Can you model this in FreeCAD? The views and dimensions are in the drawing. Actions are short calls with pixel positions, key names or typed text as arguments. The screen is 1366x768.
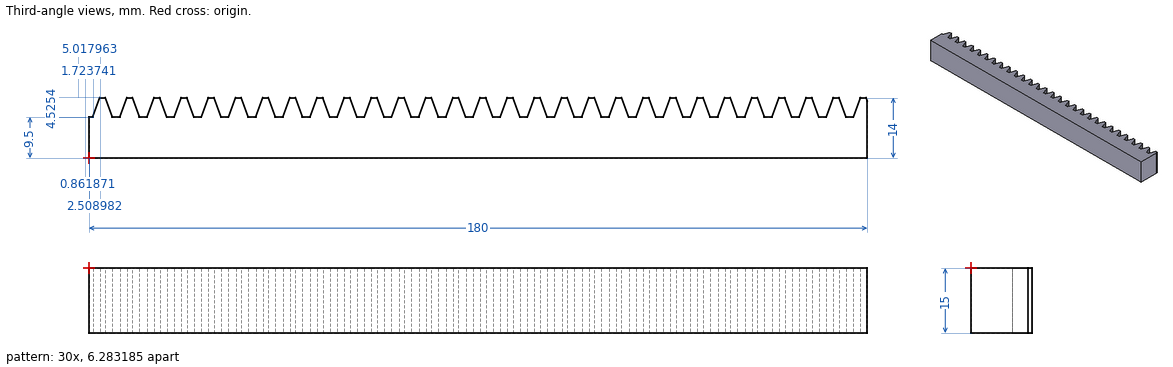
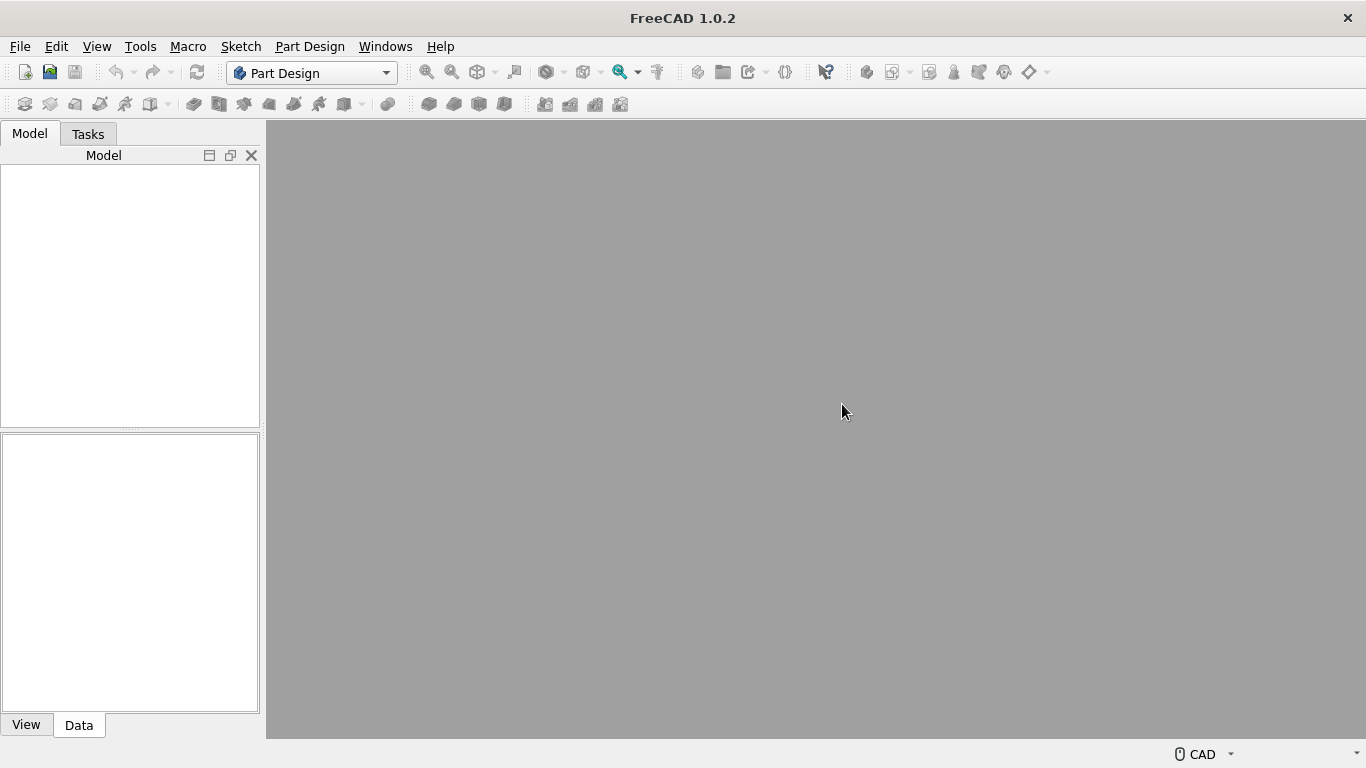
key(ctrl+n)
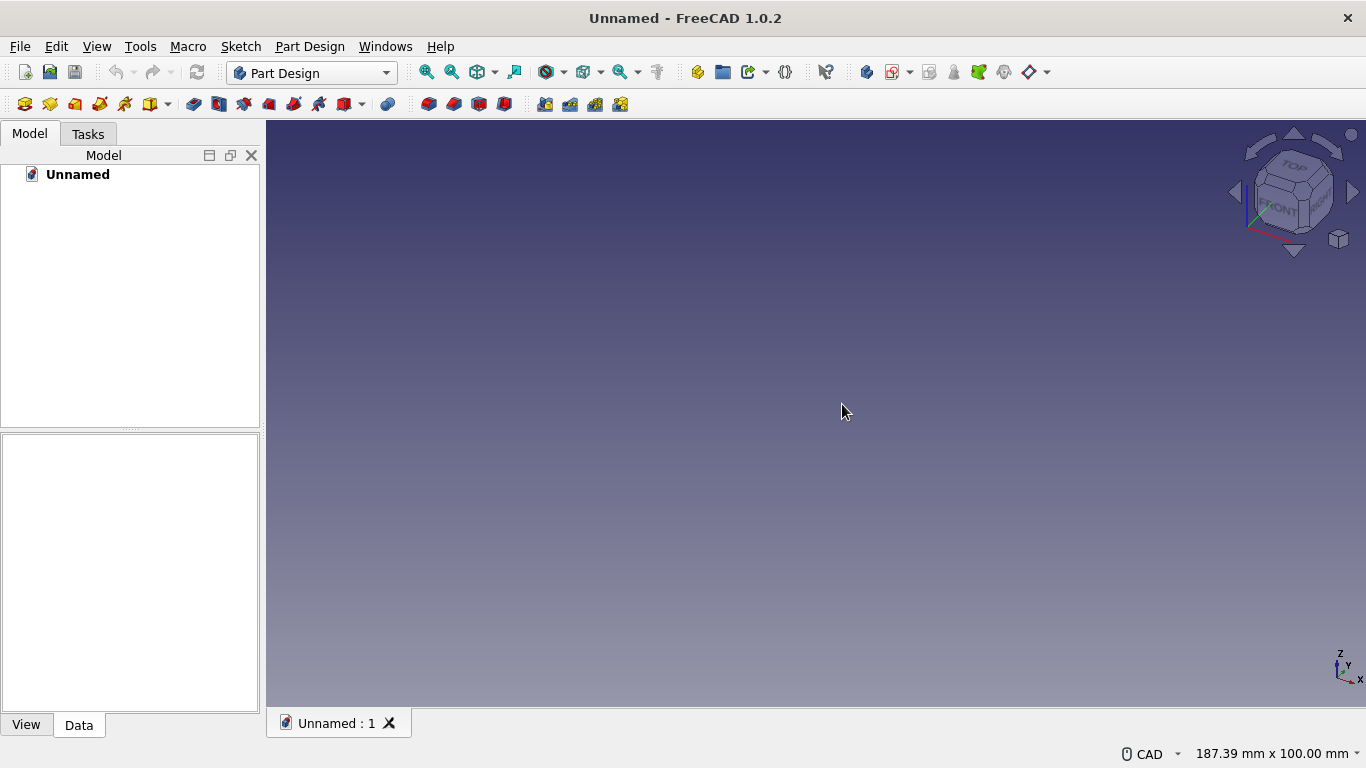
click(892, 72)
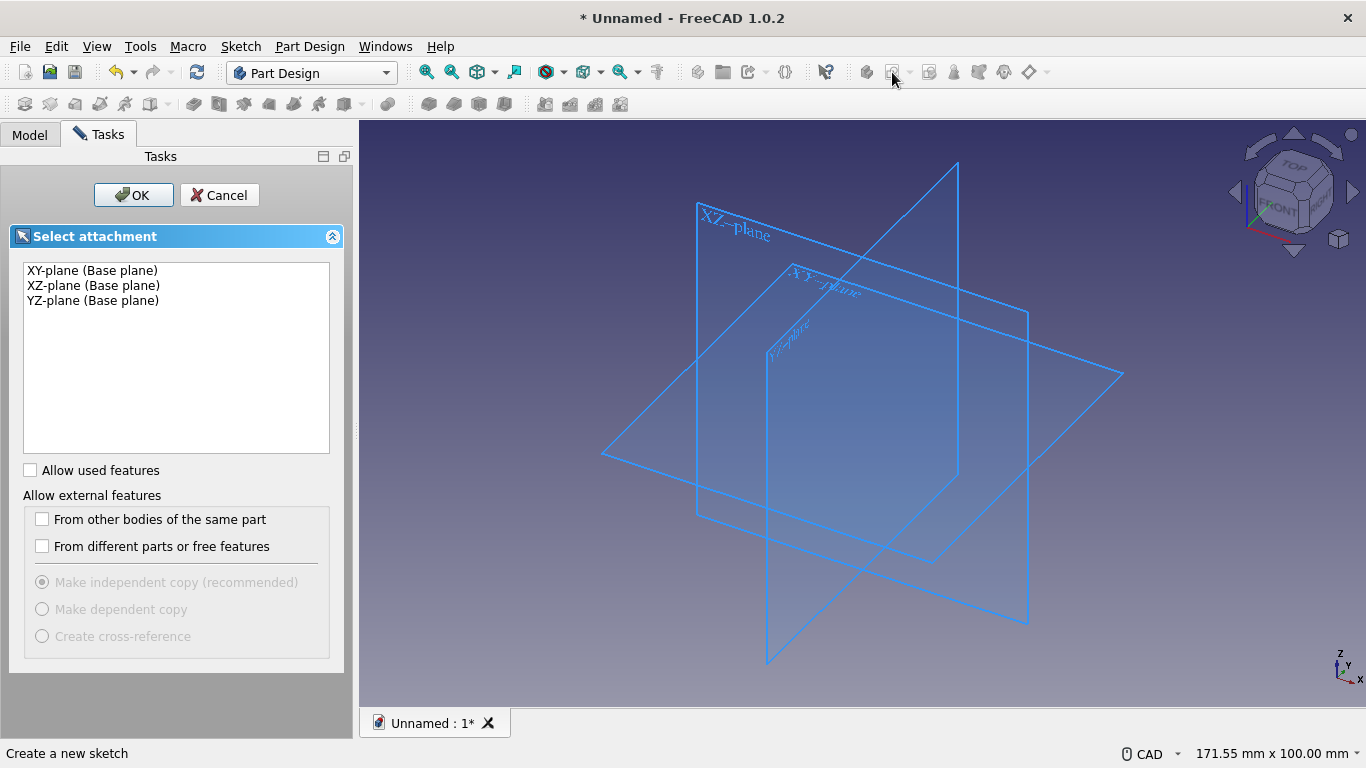
click(84, 270)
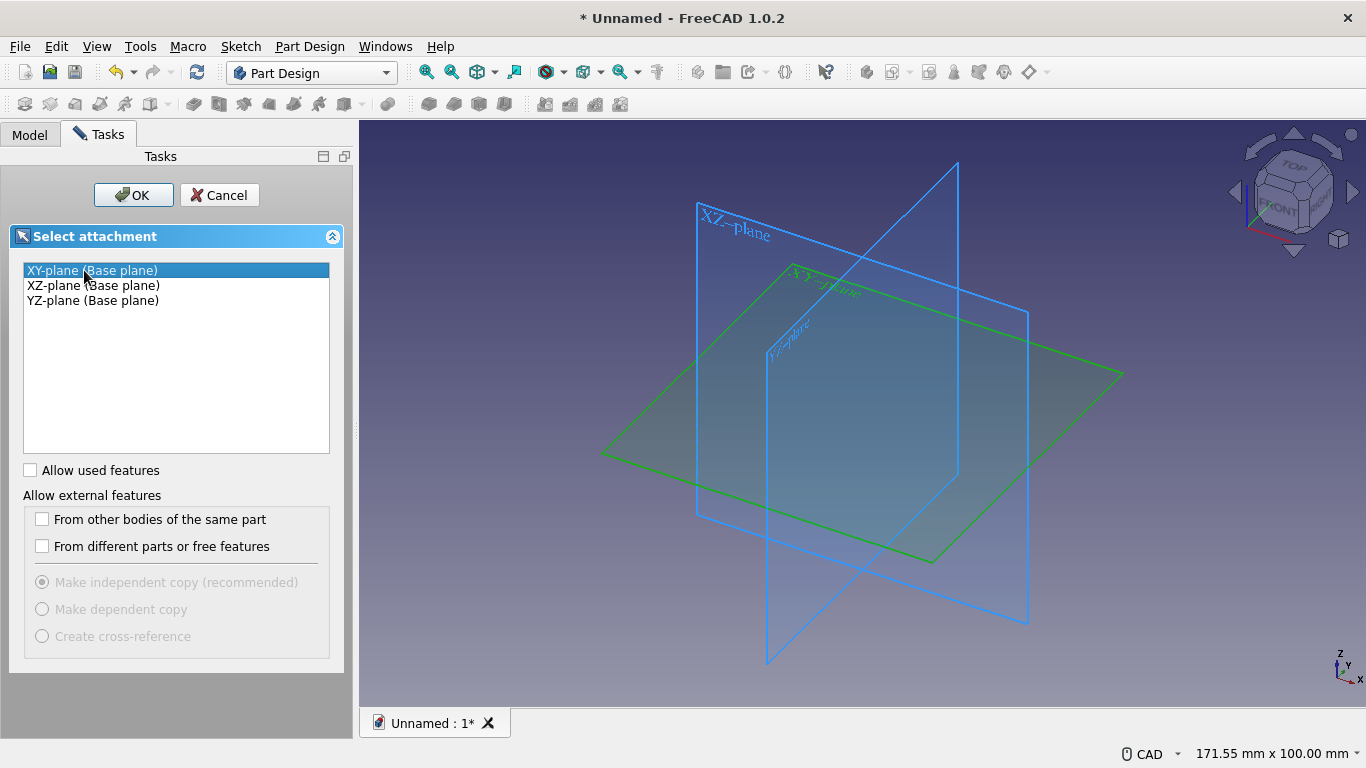
click(134, 195)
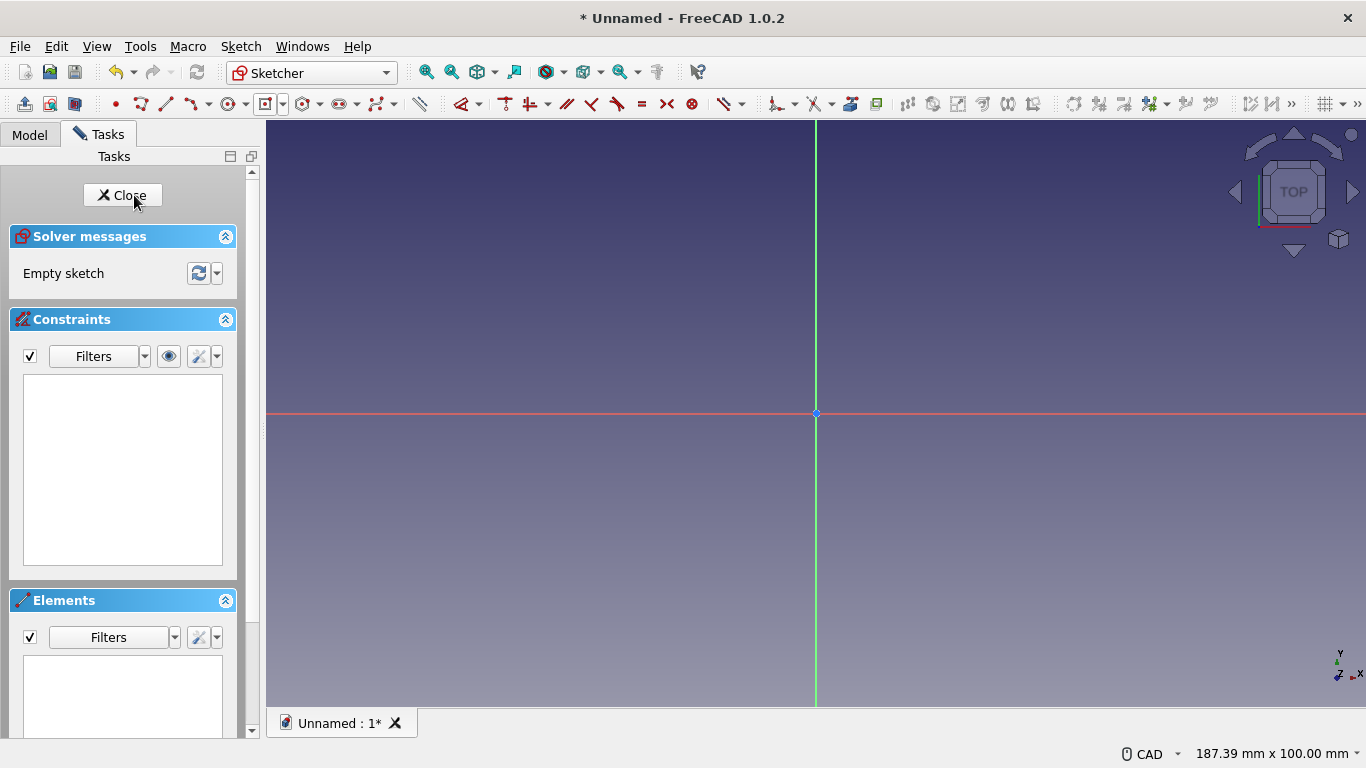
scroll(294, 463, down, 3)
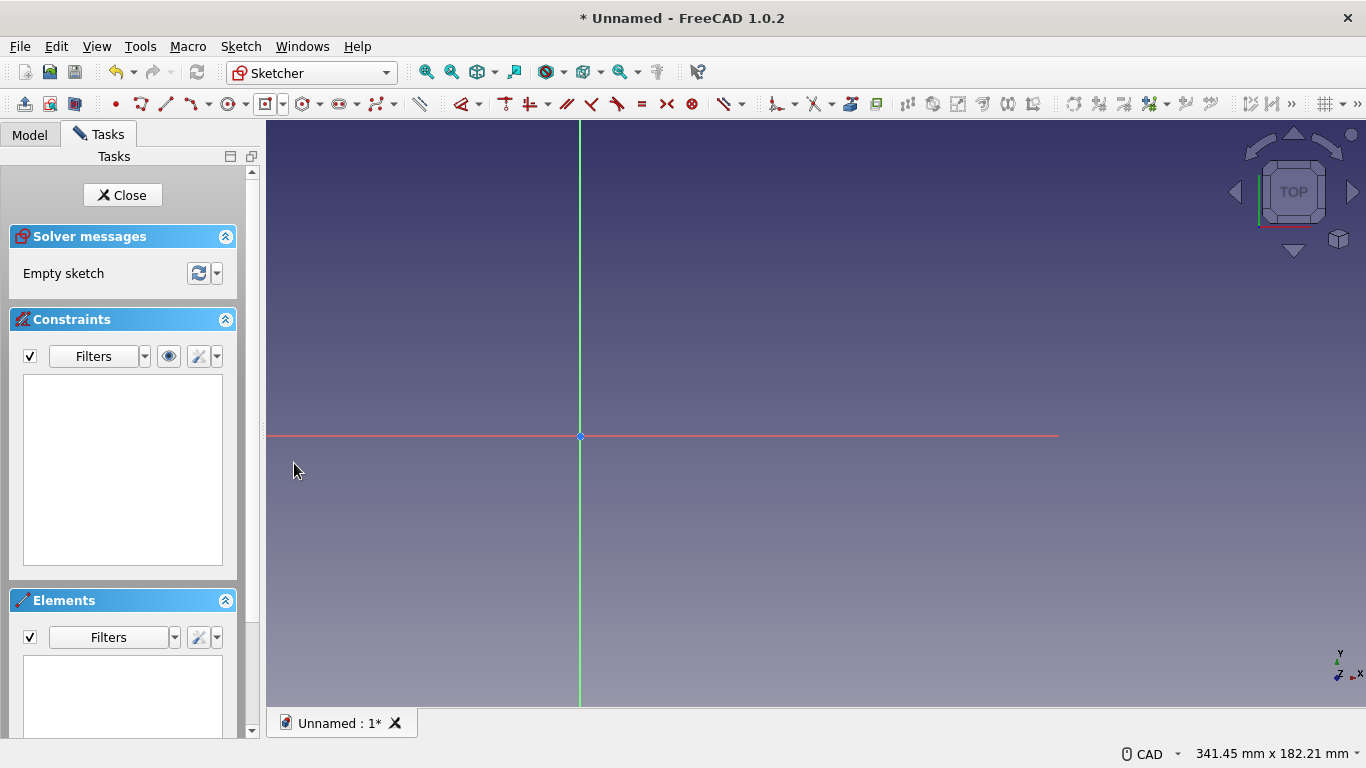
key(g)
key(r)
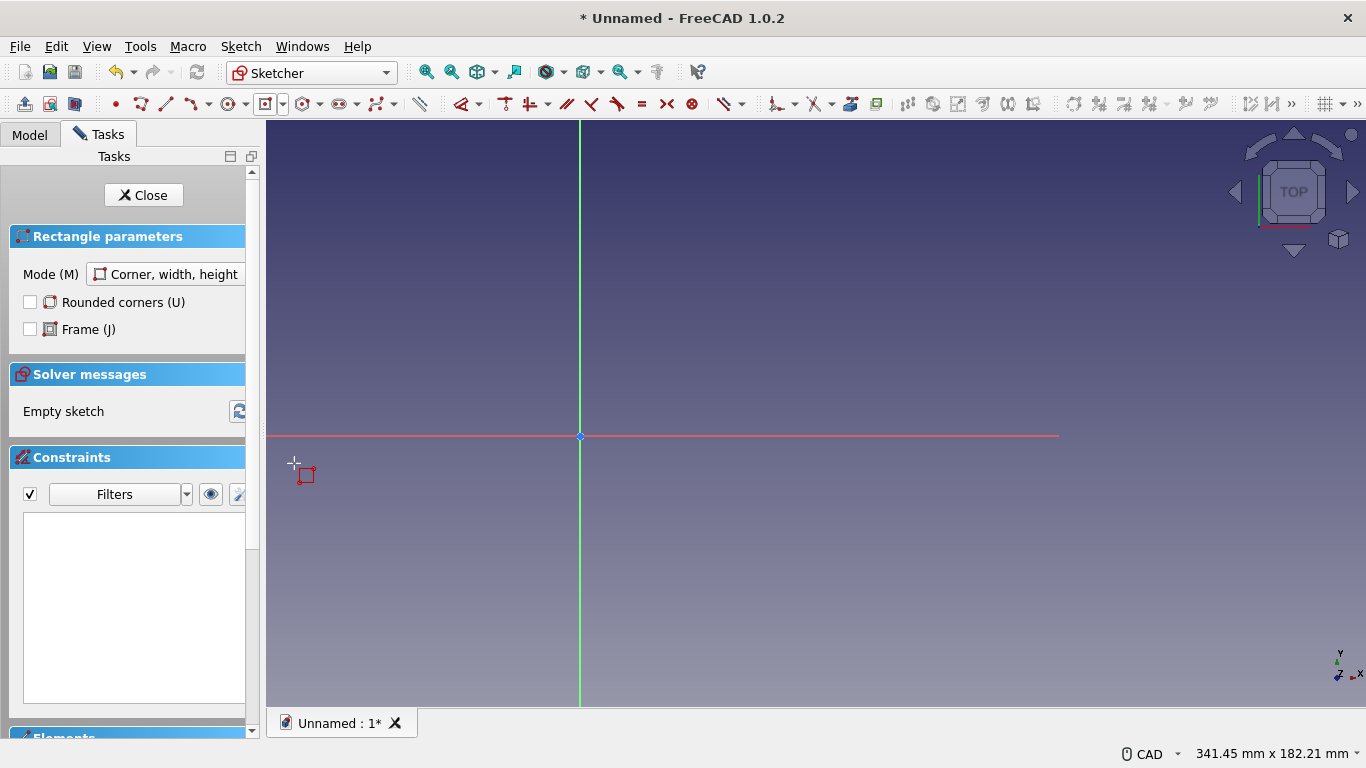
click(580, 436)
move(1160, 391)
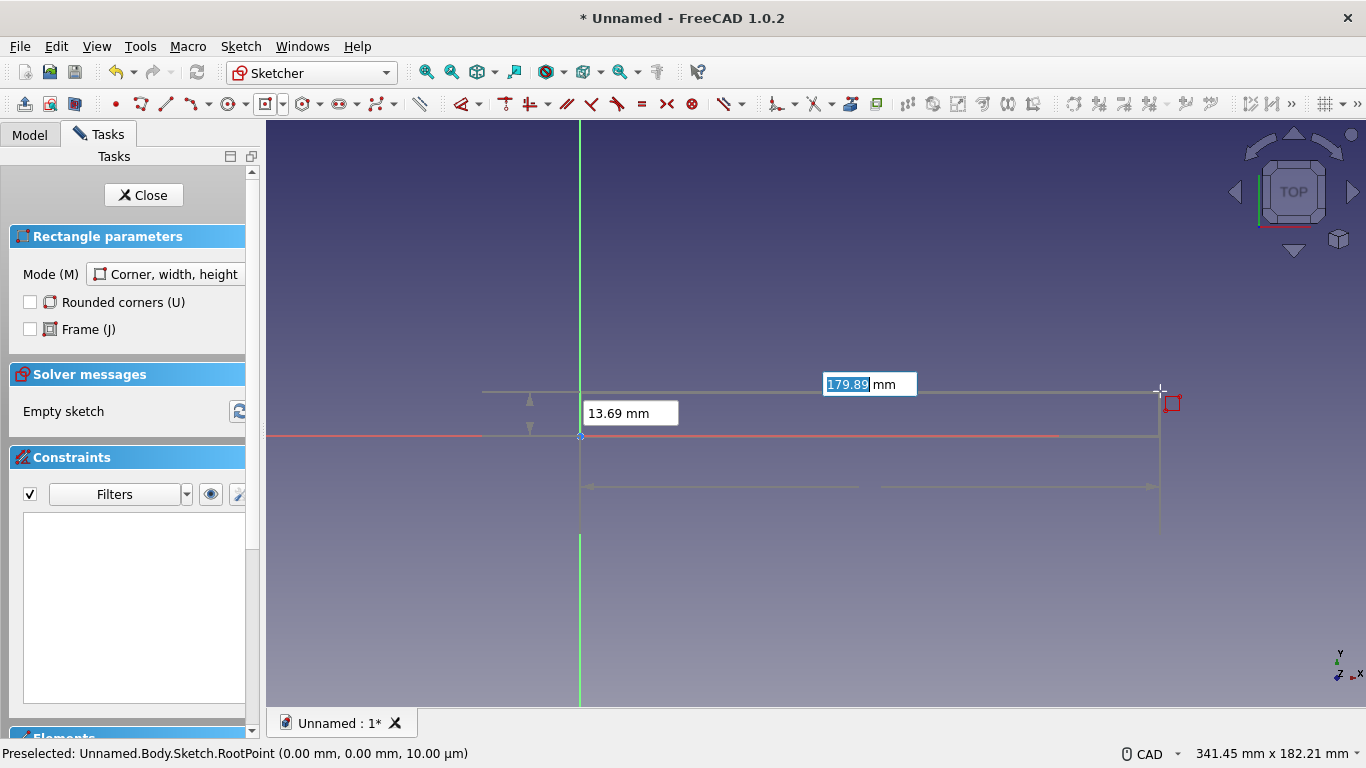
text(180)
key(Tab)
text(14)
key(Return)
key(Escape)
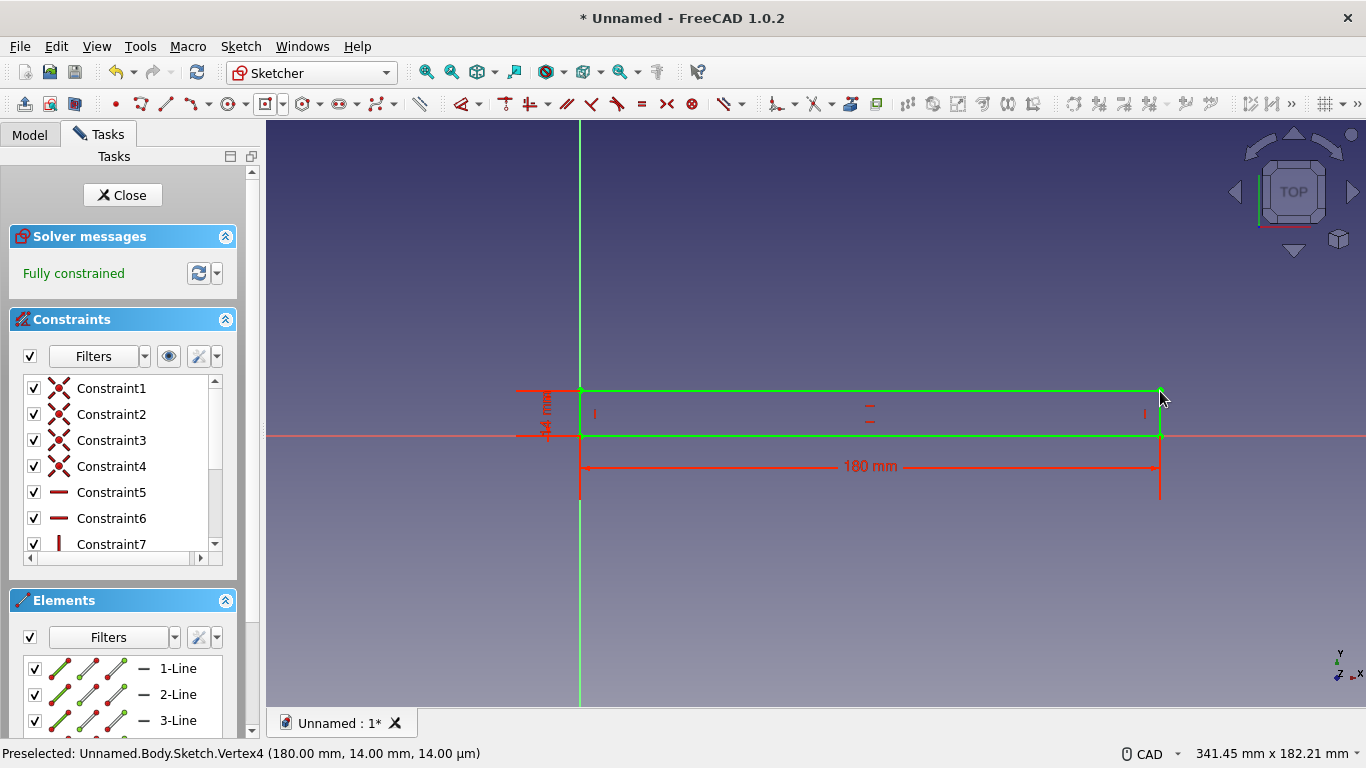
click(123, 195)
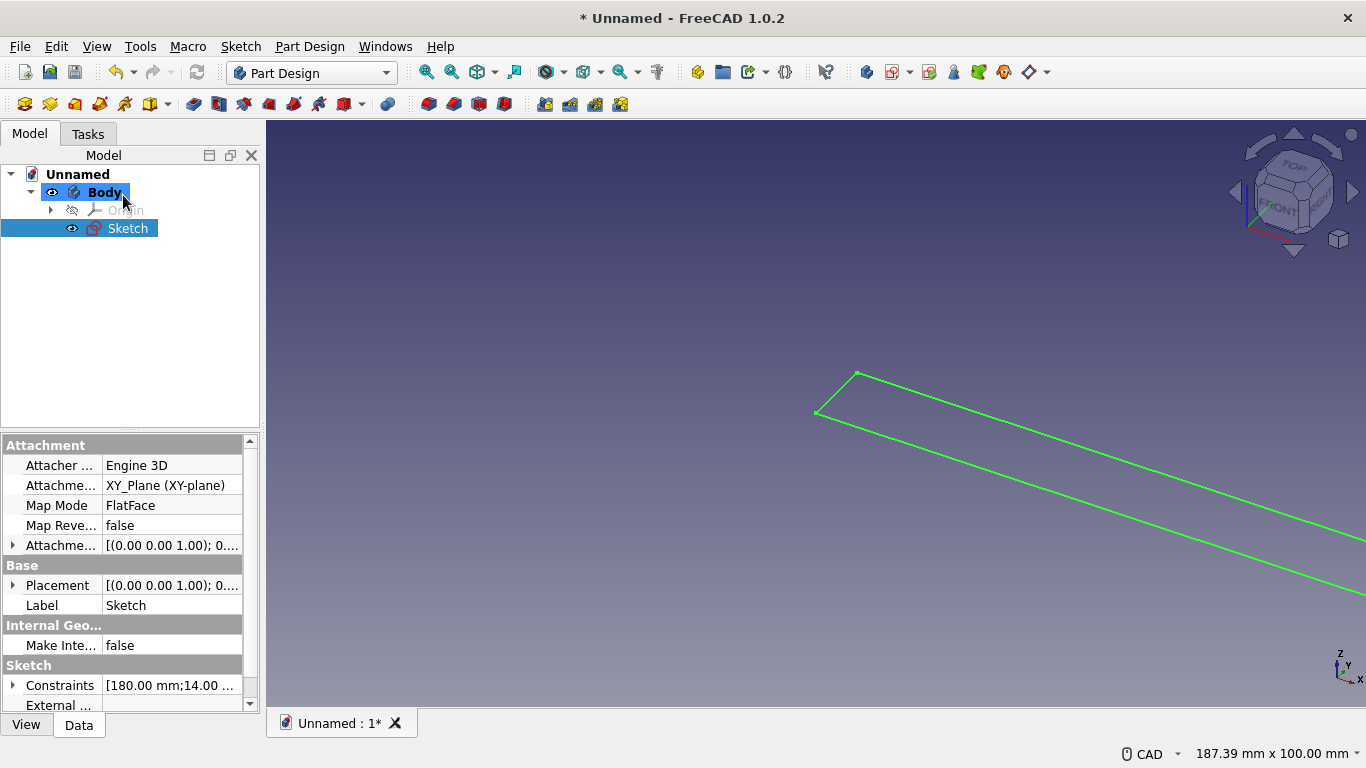
click(25, 104)